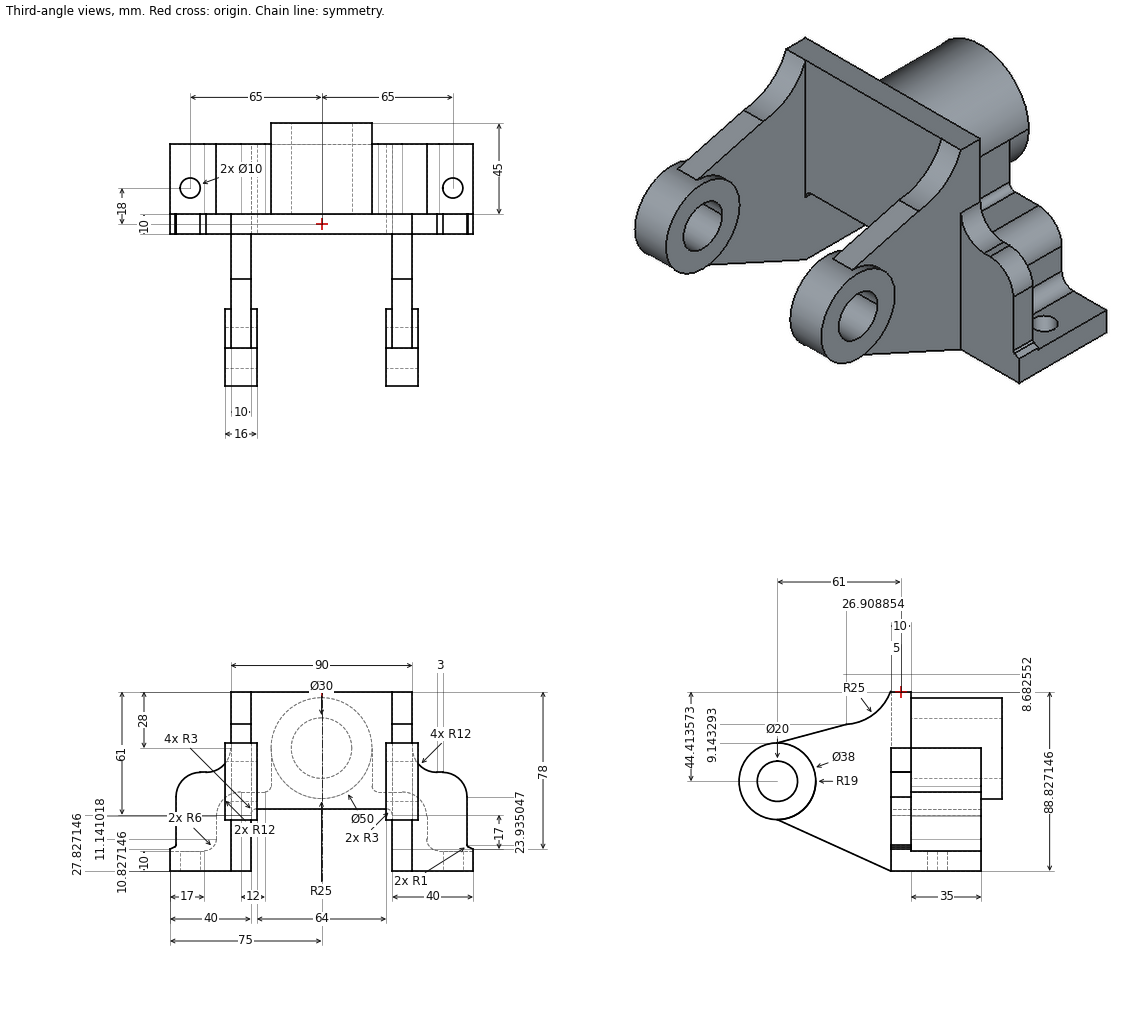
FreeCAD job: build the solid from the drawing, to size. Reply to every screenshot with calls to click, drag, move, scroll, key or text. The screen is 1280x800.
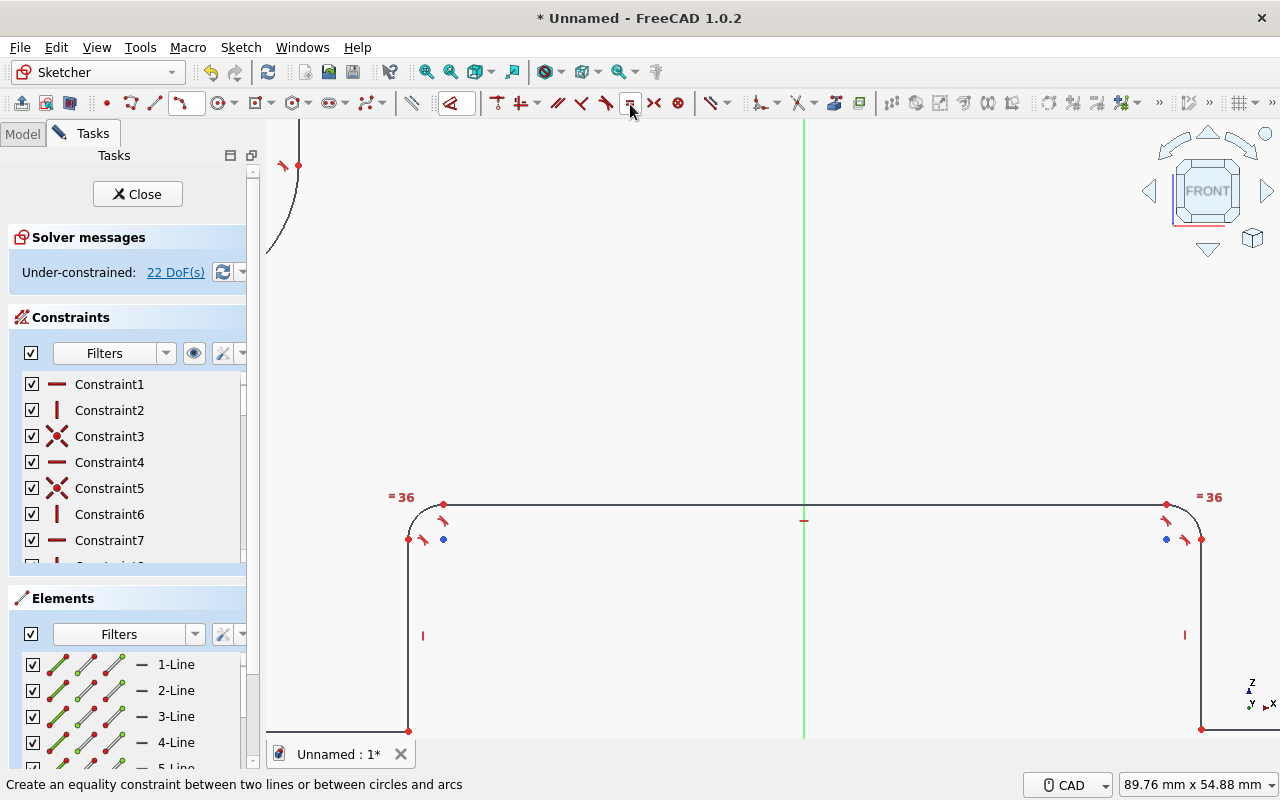
scroll(646, 511, down, 5)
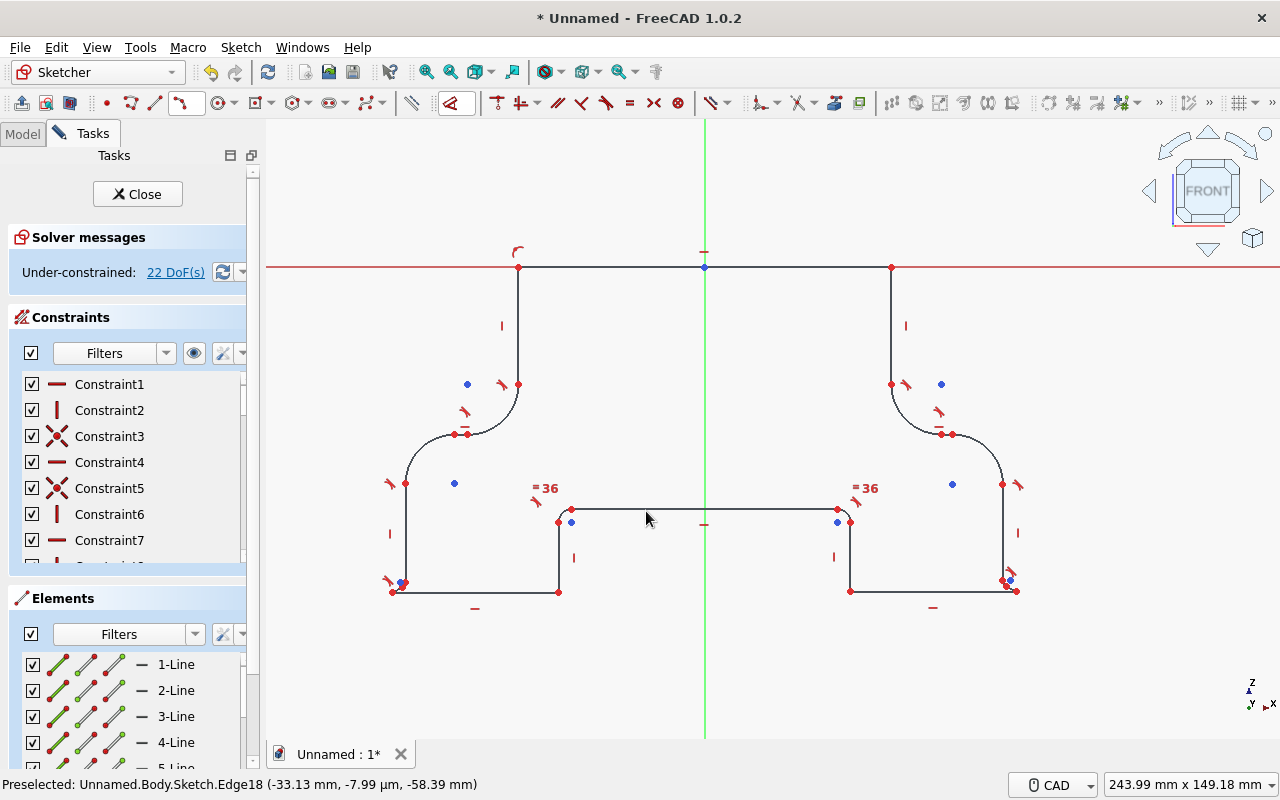
scroll(1004, 584, up, 7)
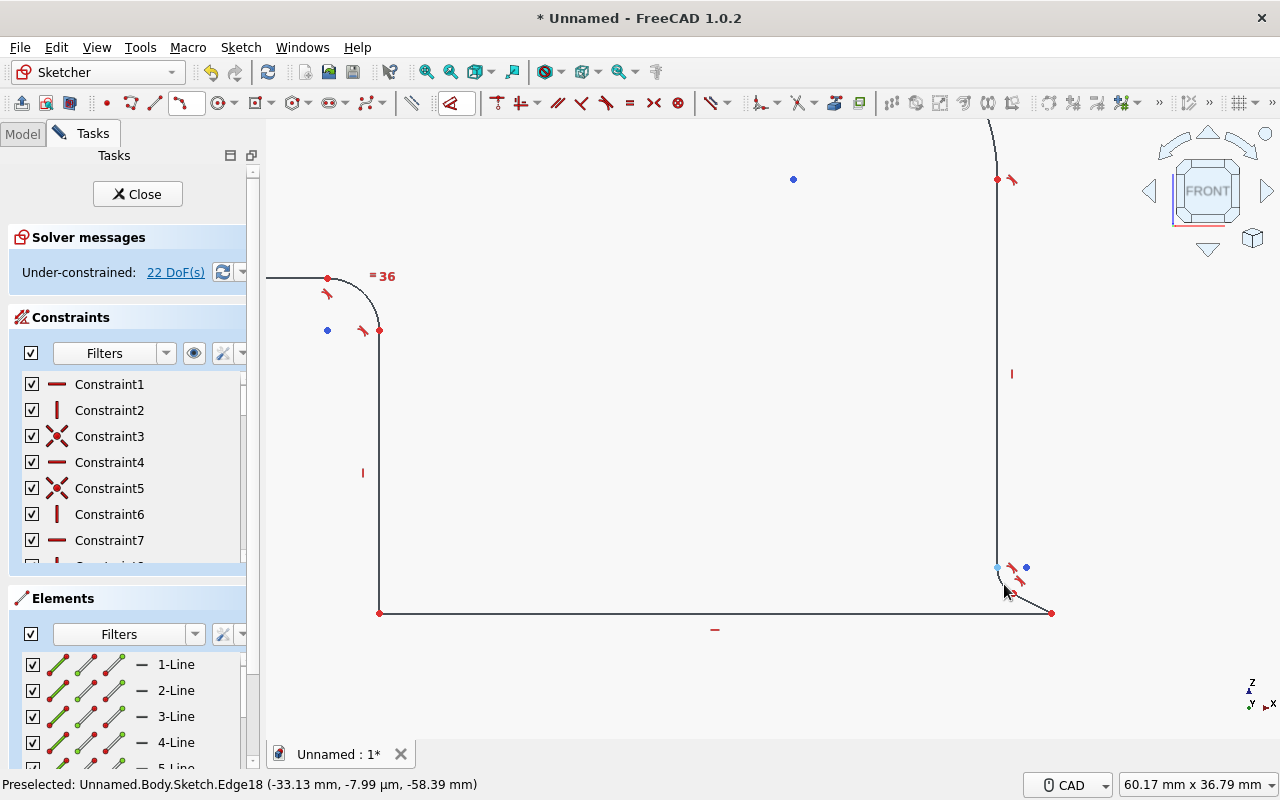
click(1002, 583)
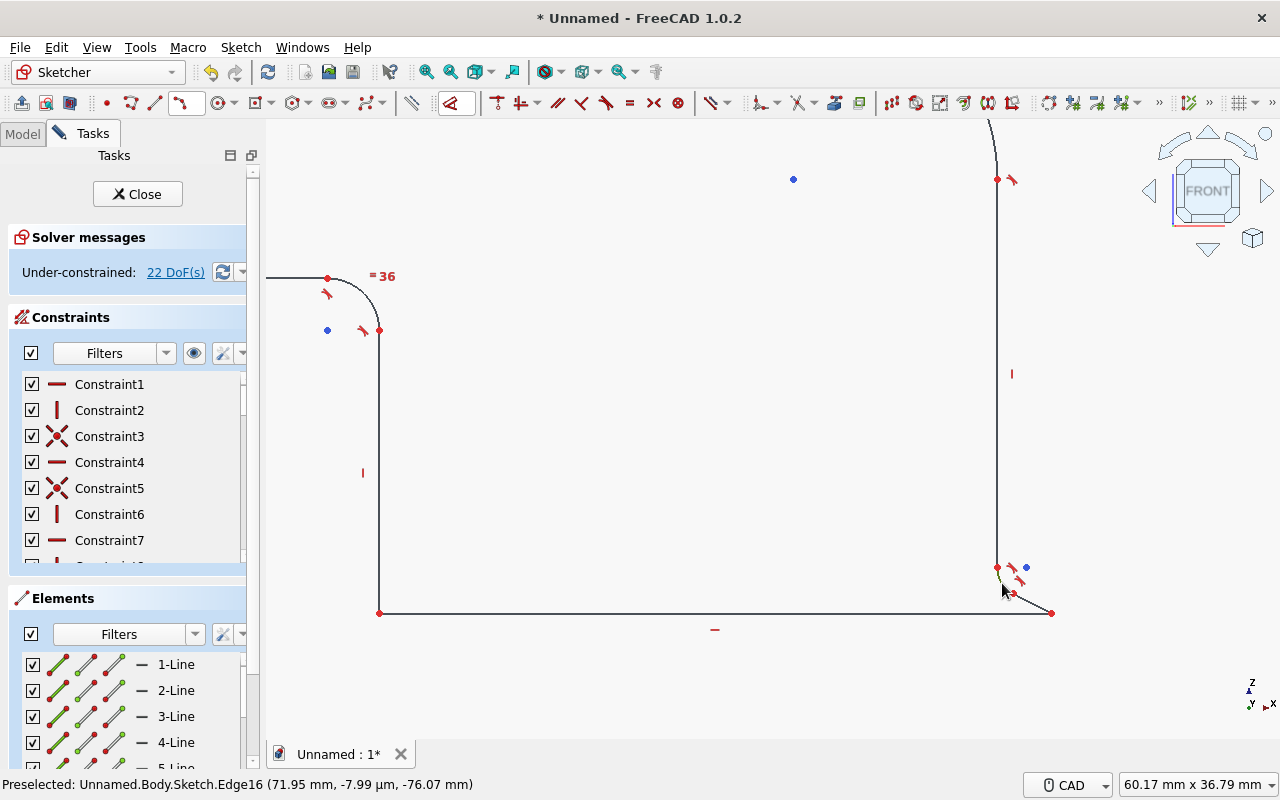
scroll(1005, 584, down, 7)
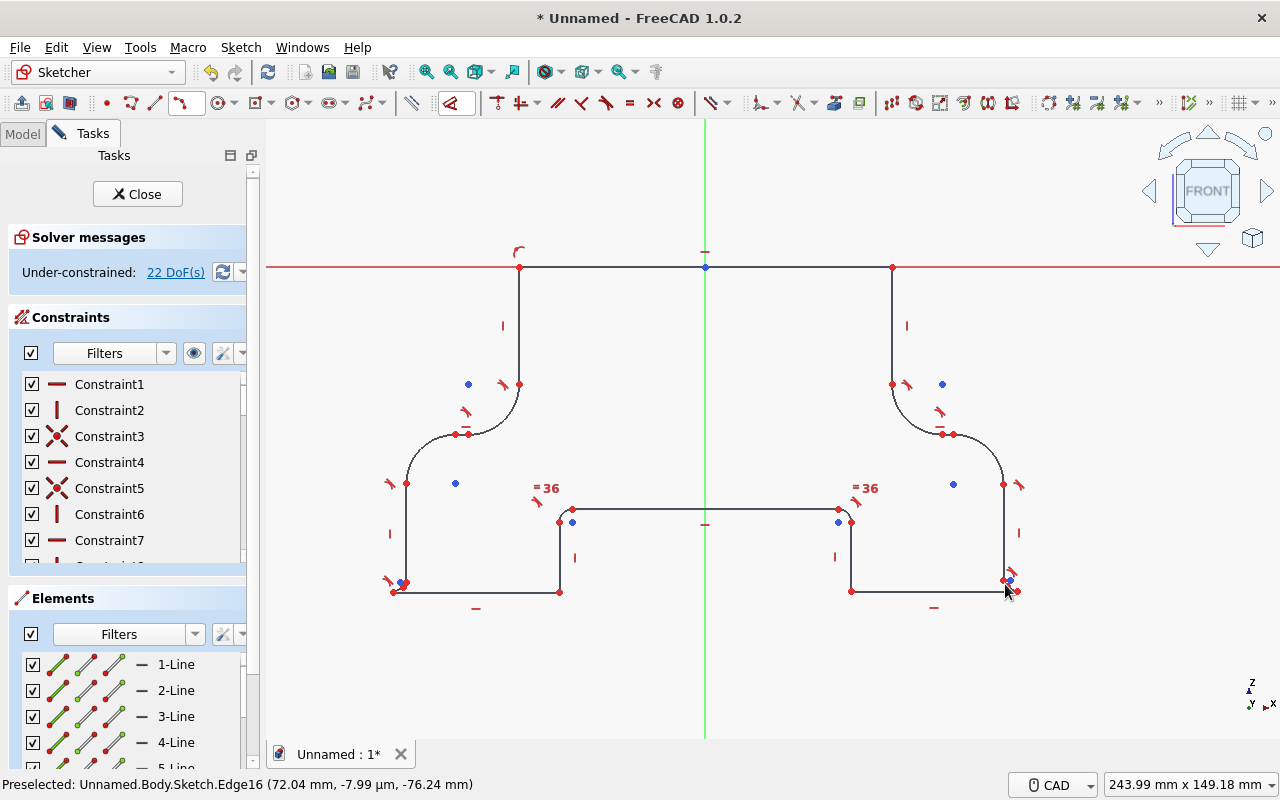
scroll(406, 585, up, 8)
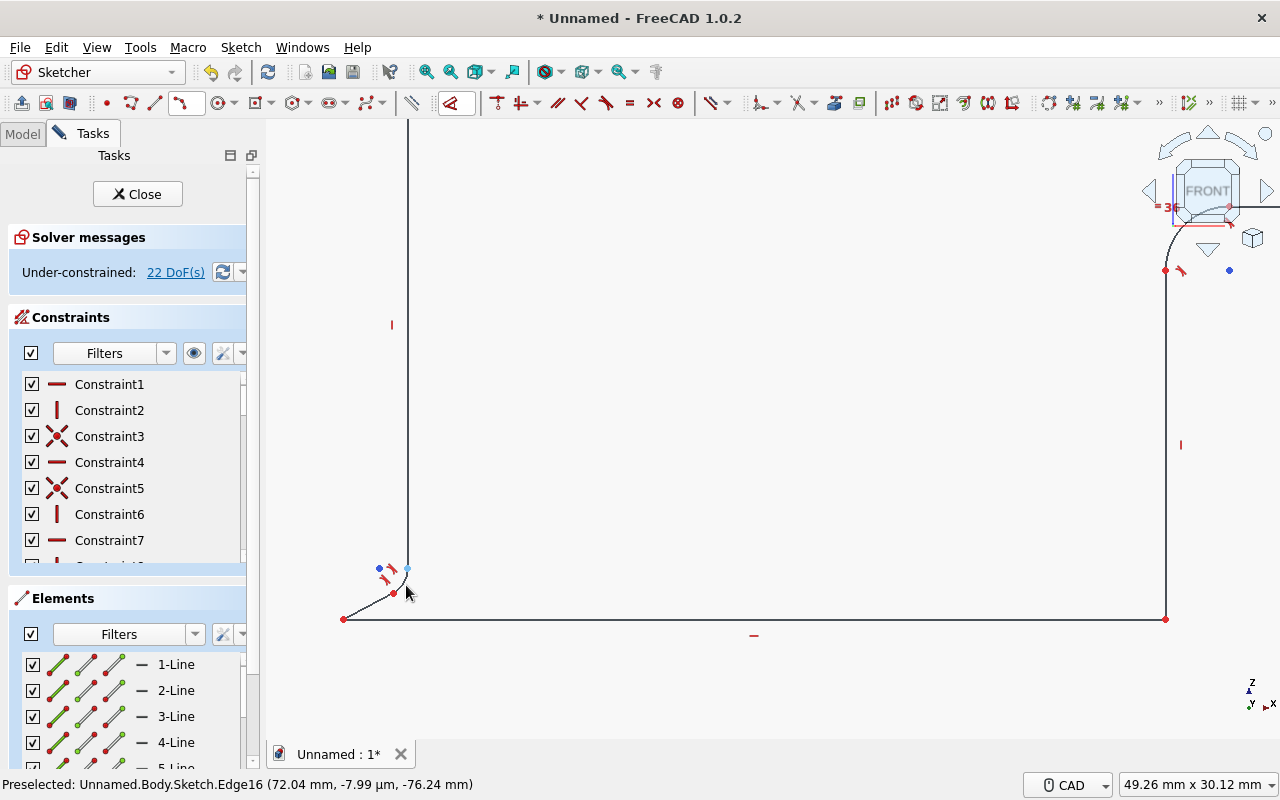
click(404, 583)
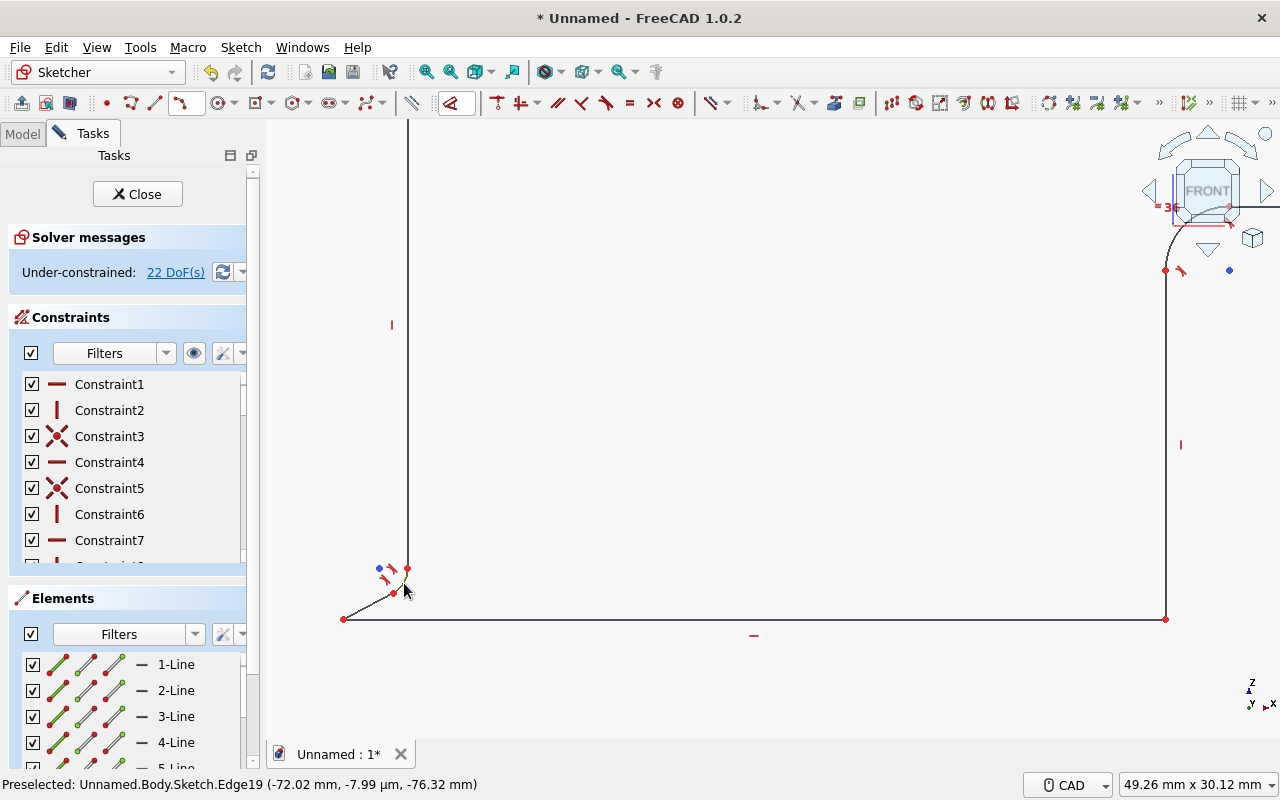
key(e)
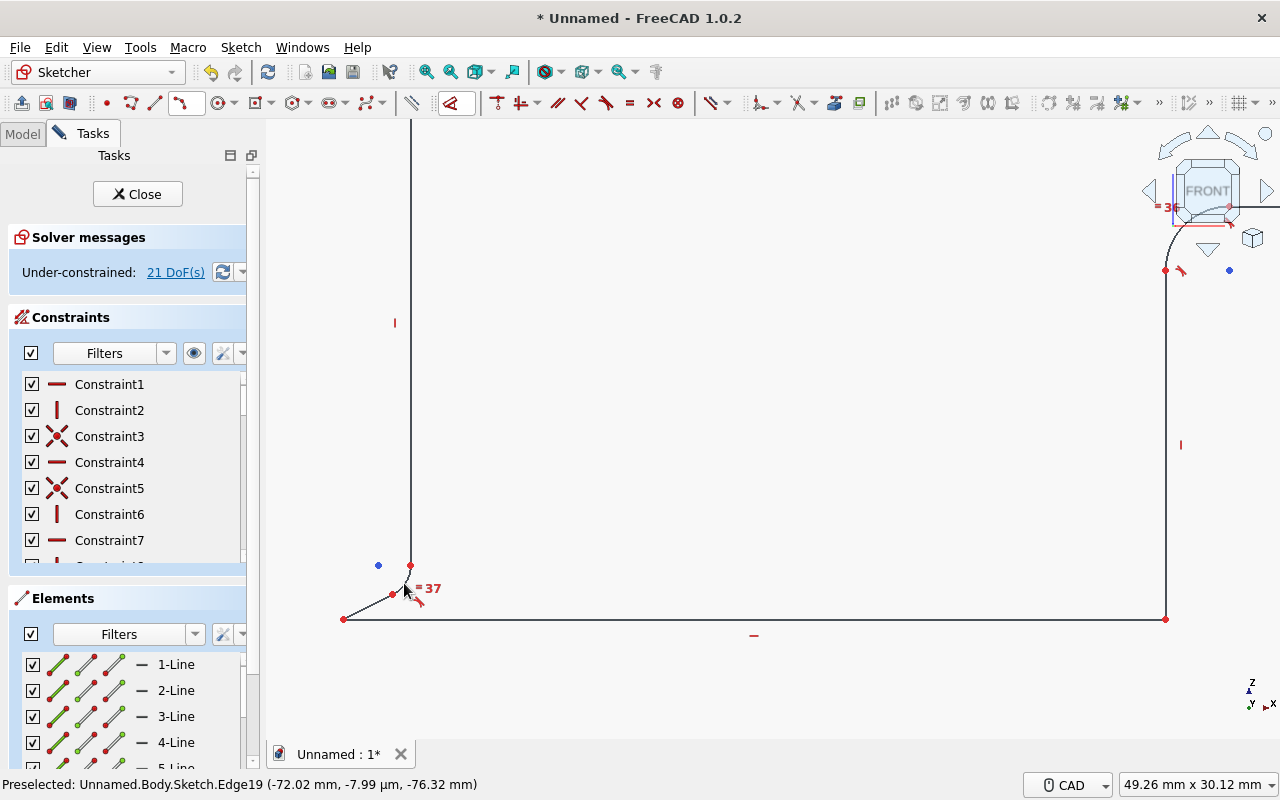
scroll(405, 585, down, 8)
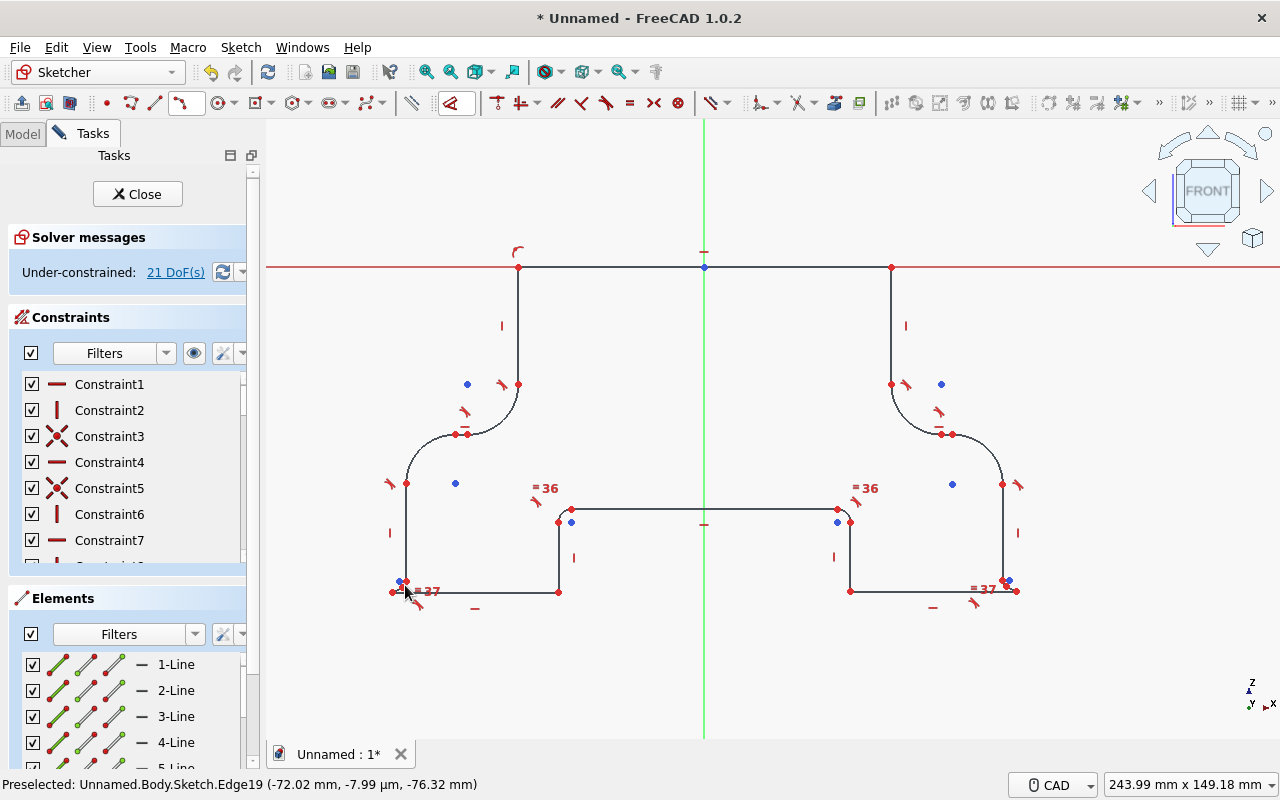
click(997, 462)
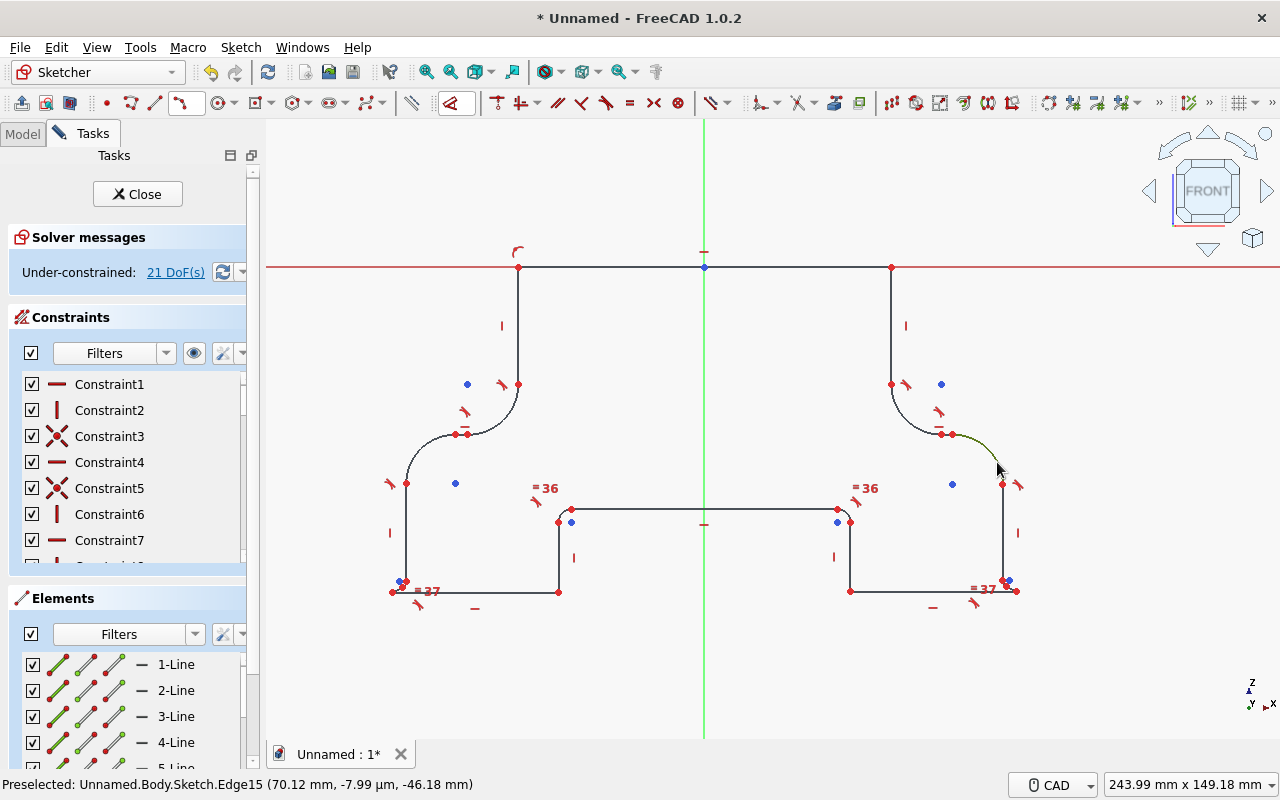
click(433, 440)